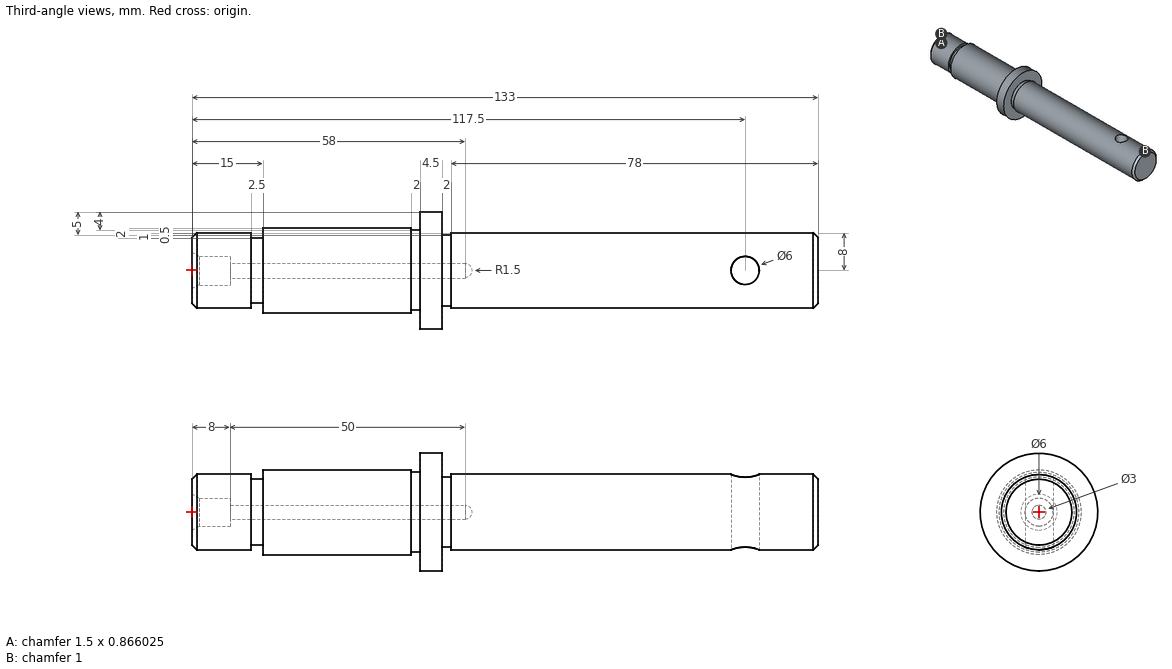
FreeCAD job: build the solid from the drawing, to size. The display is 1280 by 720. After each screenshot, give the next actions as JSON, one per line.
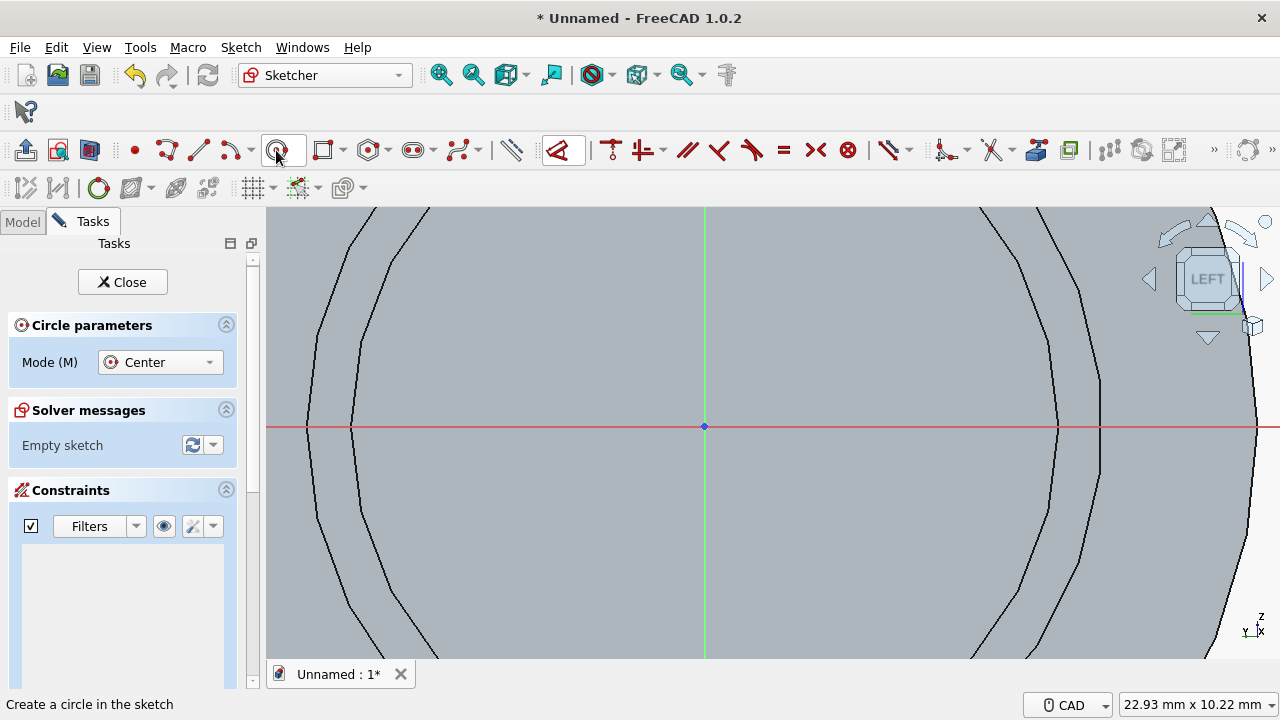
{"action": "left_click", "coordinate": [705, 427]}
{"action": "mouse_move", "coordinate": [798, 333]}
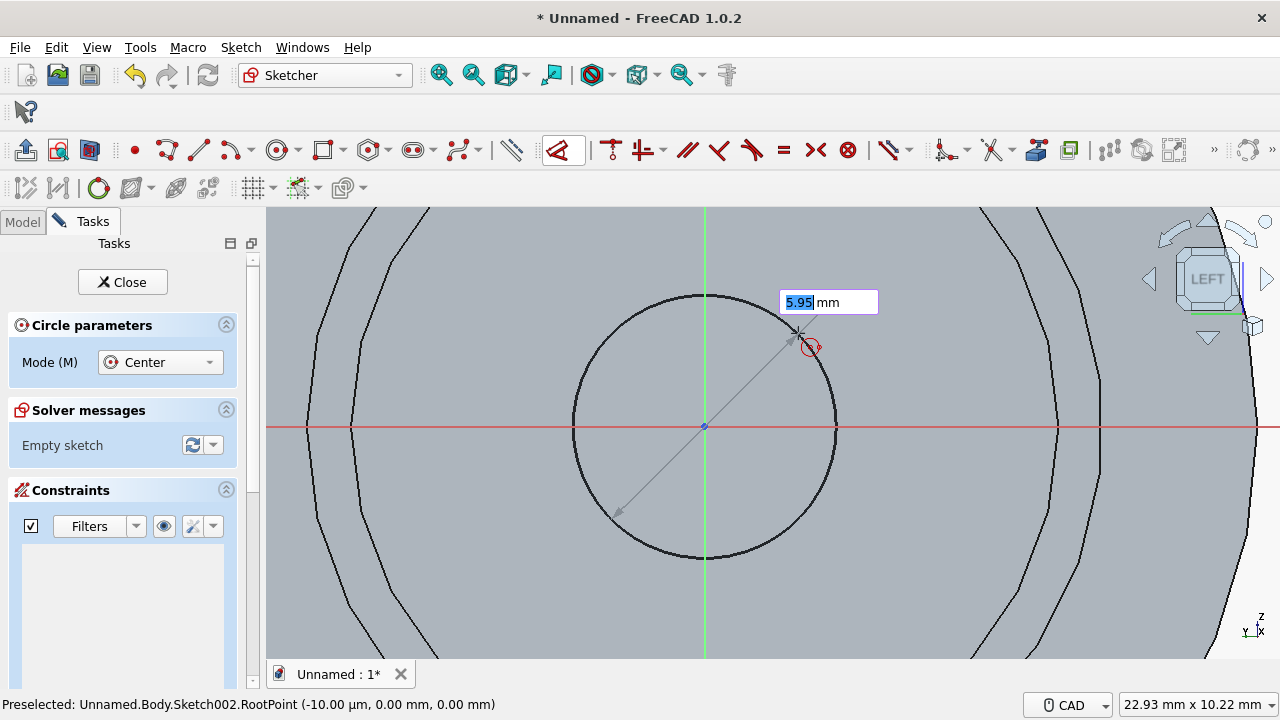
{"action": "type", "text": "6"}
{"action": "key", "text": "Return"}
{"action": "key", "text": "Escape"}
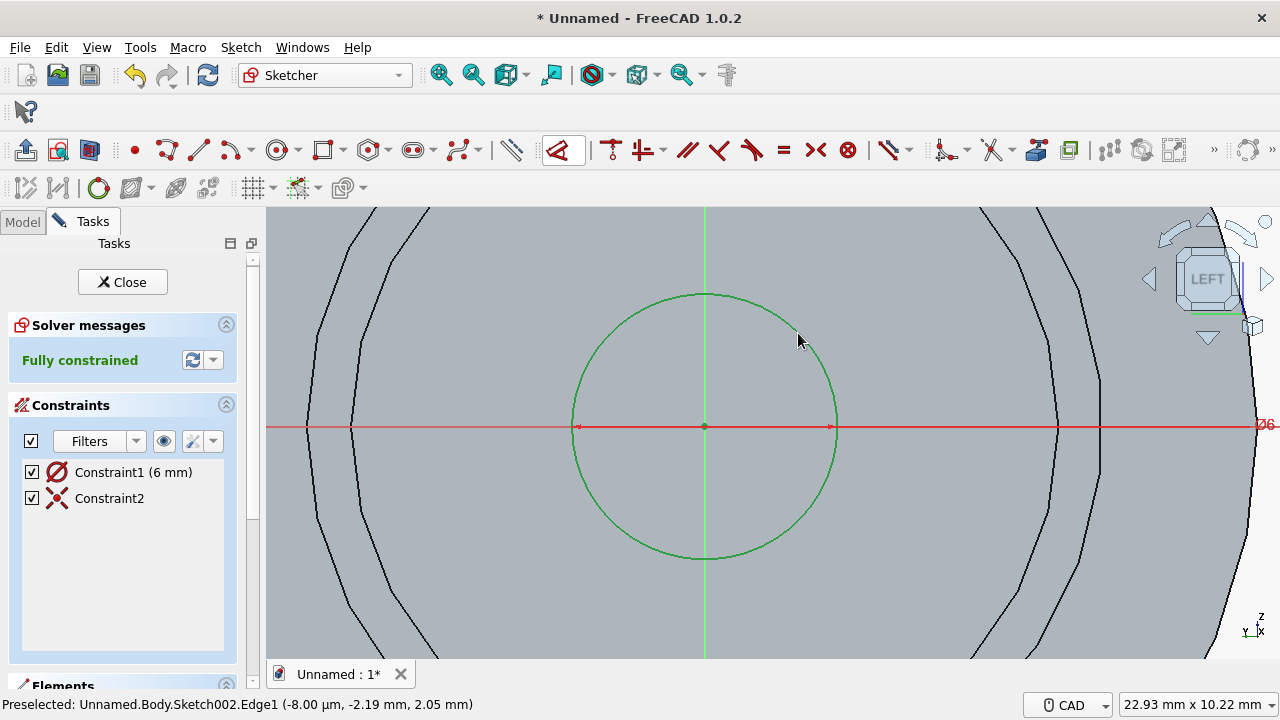
{"action": "left_click", "coordinate": [123, 282]}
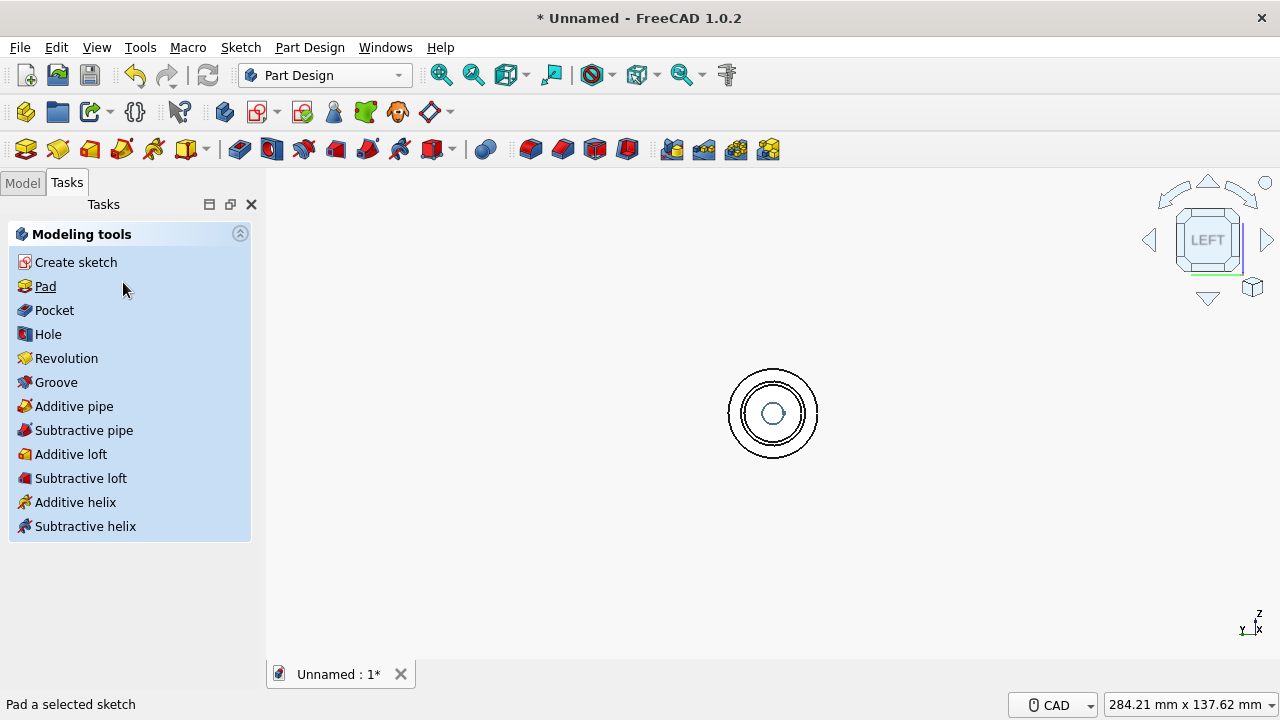
{"action": "left_click", "coordinate": [240, 150]}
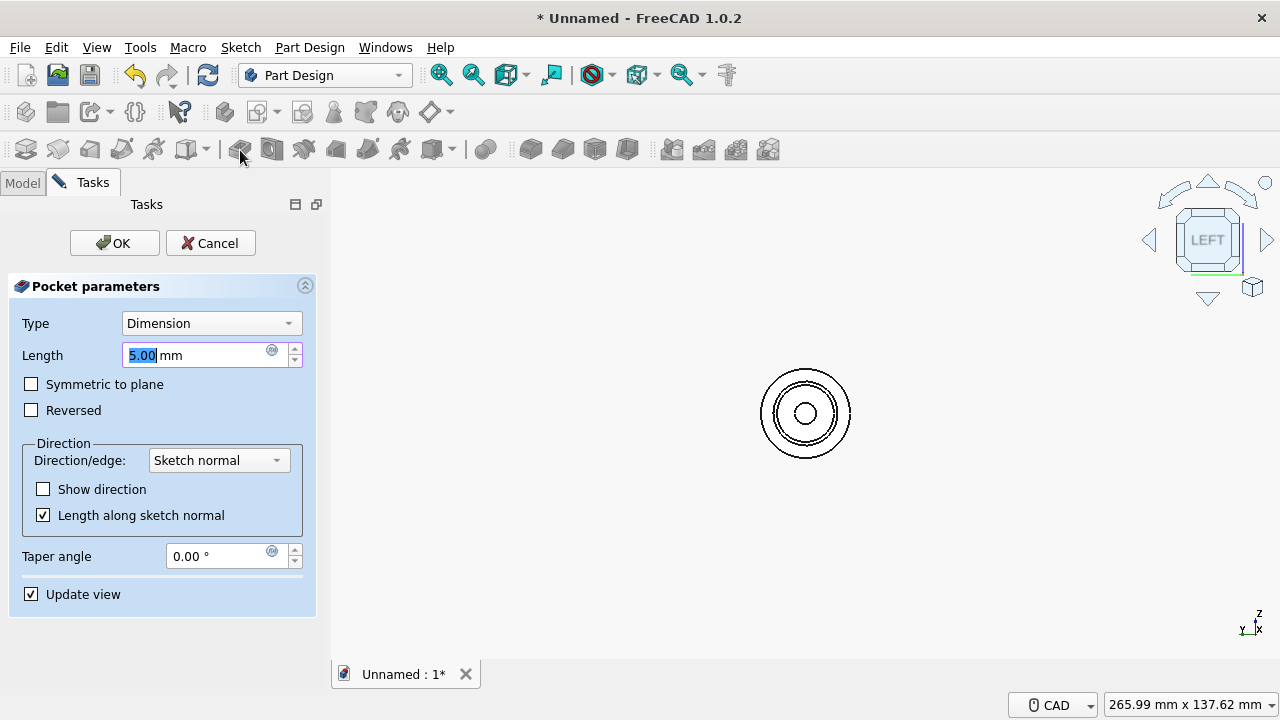
{"action": "left_click", "coordinate": [212, 324]}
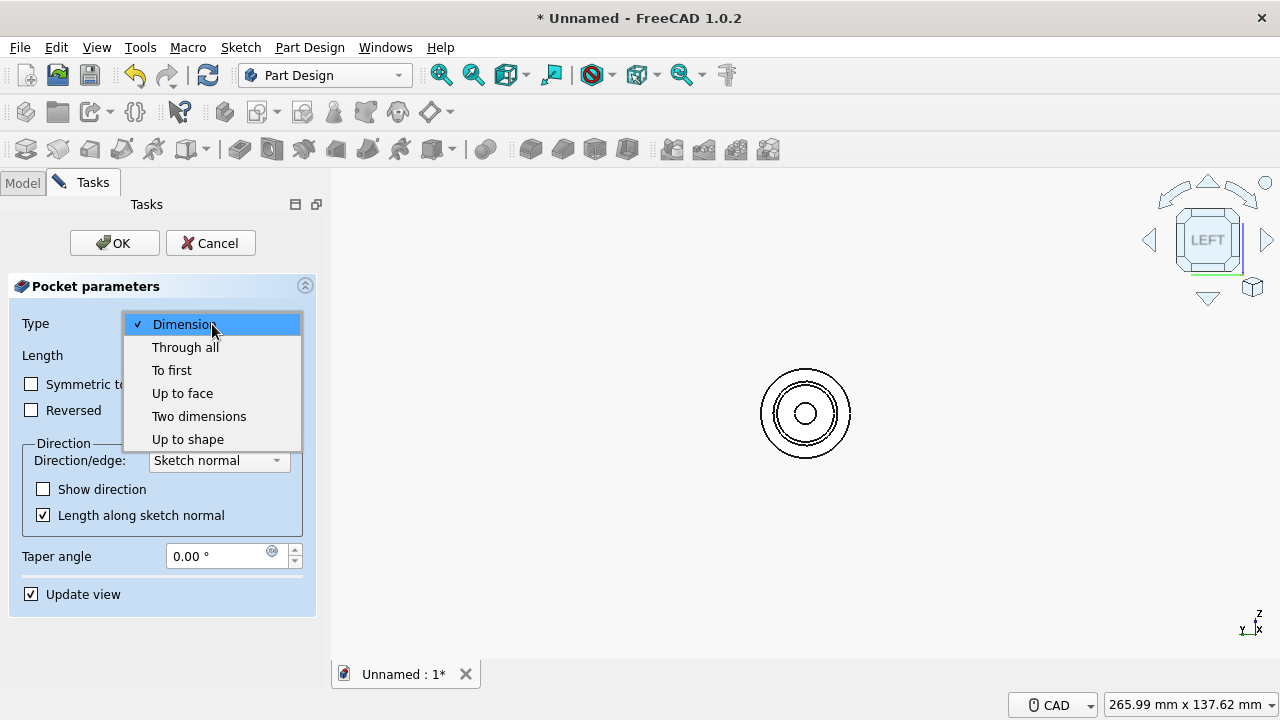
{"action": "left_click", "coordinate": [212, 416]}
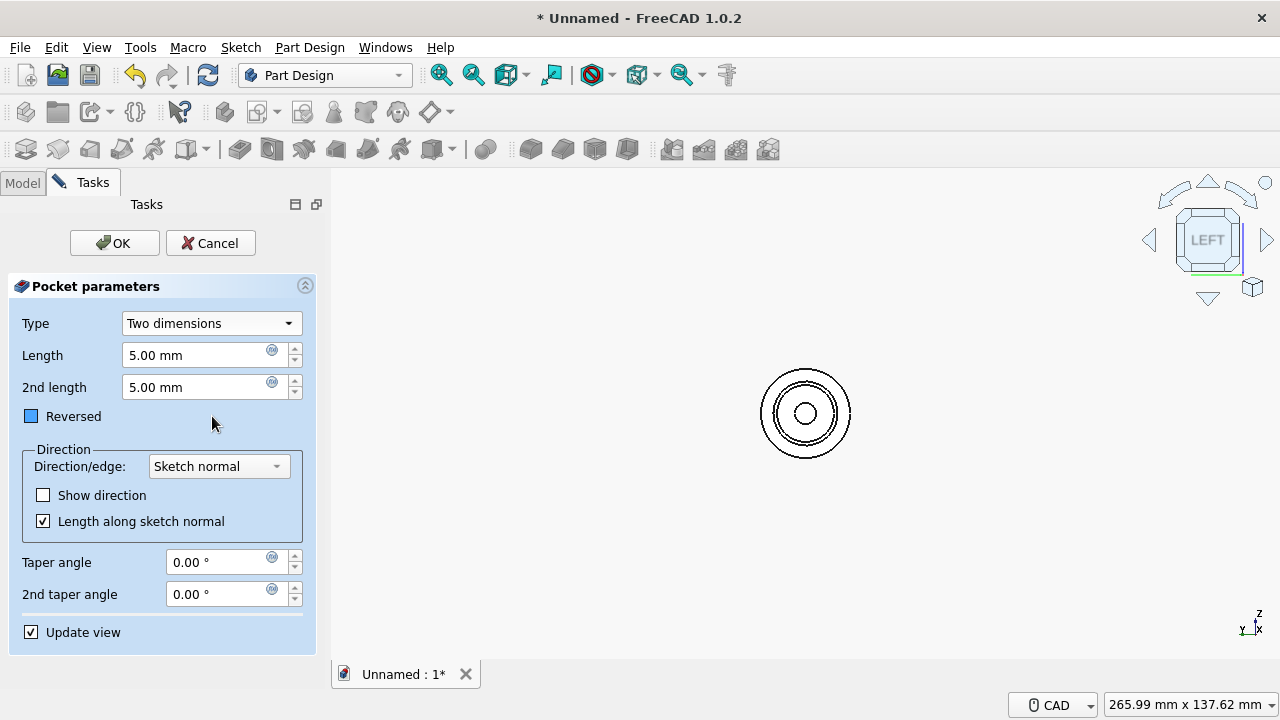
{"action": "triple_click", "coordinate": [204, 355]}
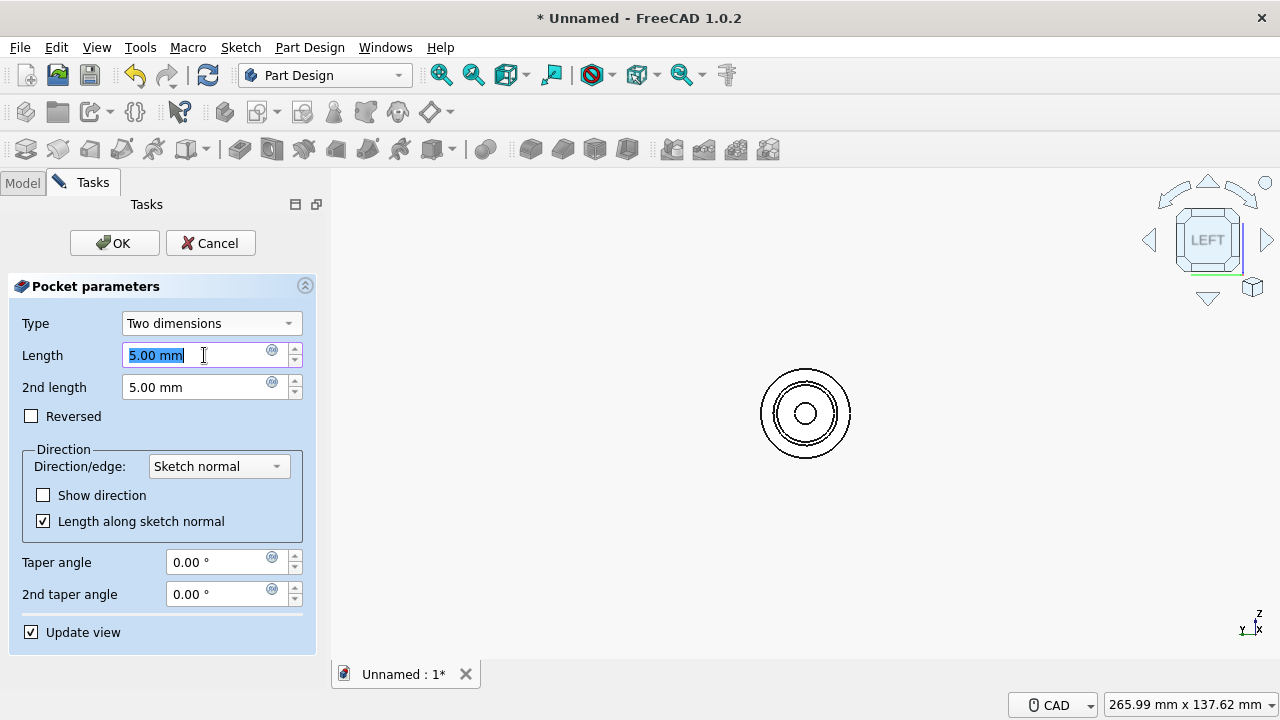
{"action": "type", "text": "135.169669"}
{"action": "key", "text": "Tab"}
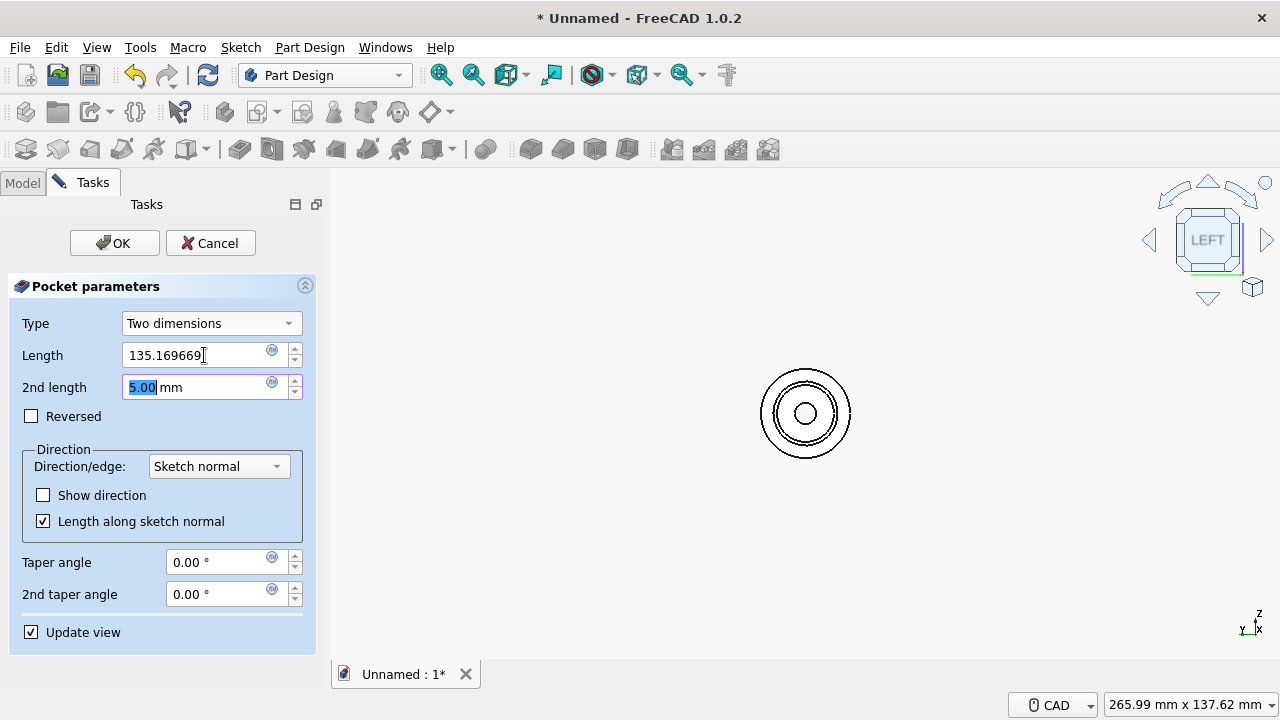
{"action": "type", "text": "8"}
{"action": "key", "text": "Tab"}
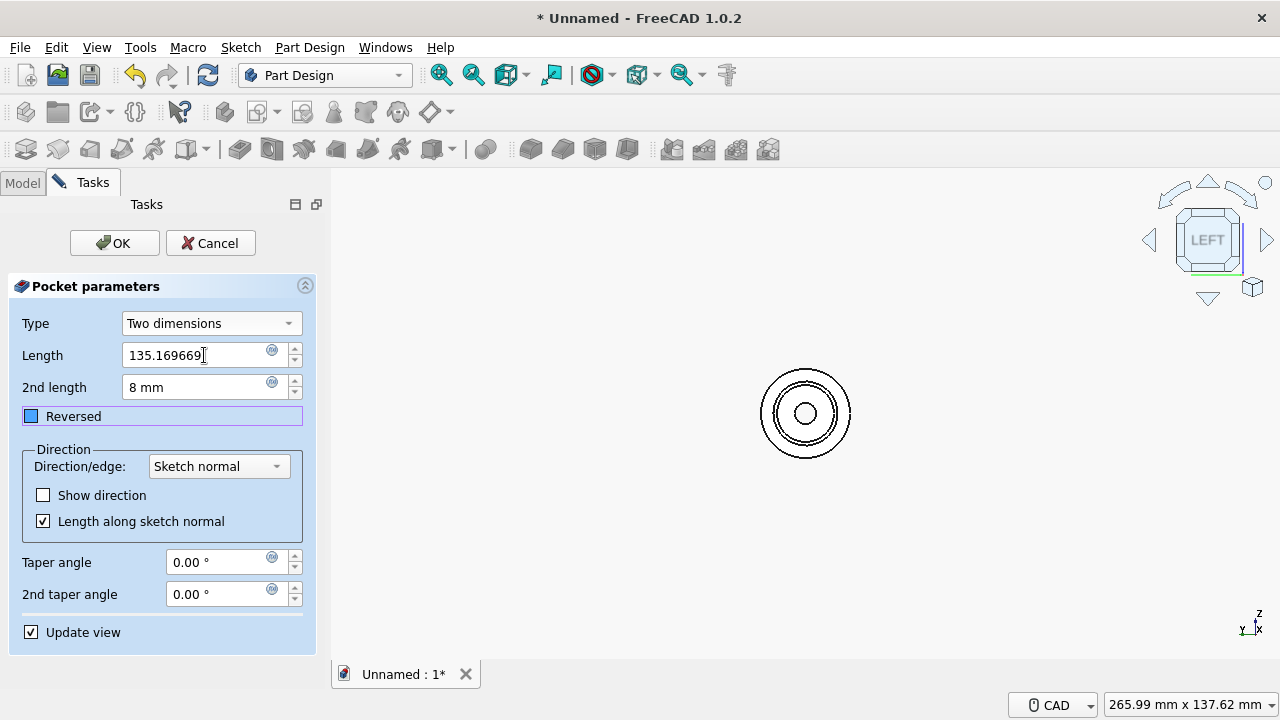
{"action": "left_click", "coordinate": [30, 416]}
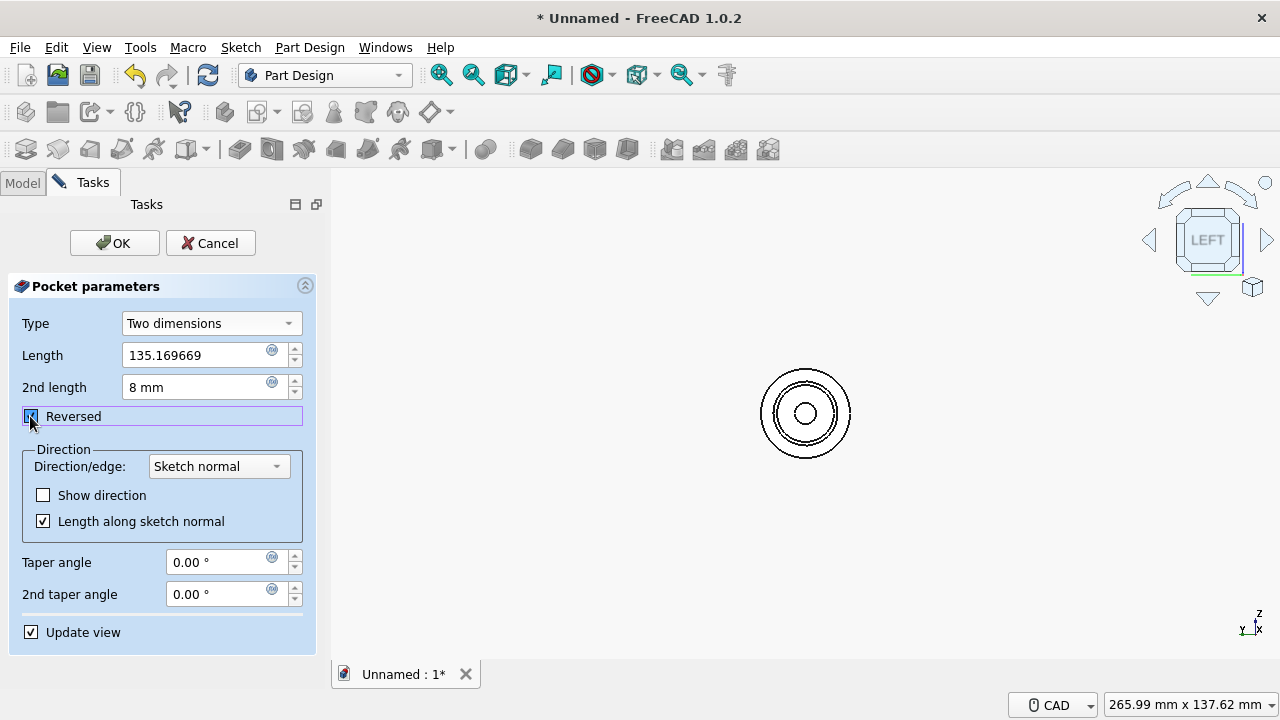
{"action": "left_click", "coordinate": [115, 243]}